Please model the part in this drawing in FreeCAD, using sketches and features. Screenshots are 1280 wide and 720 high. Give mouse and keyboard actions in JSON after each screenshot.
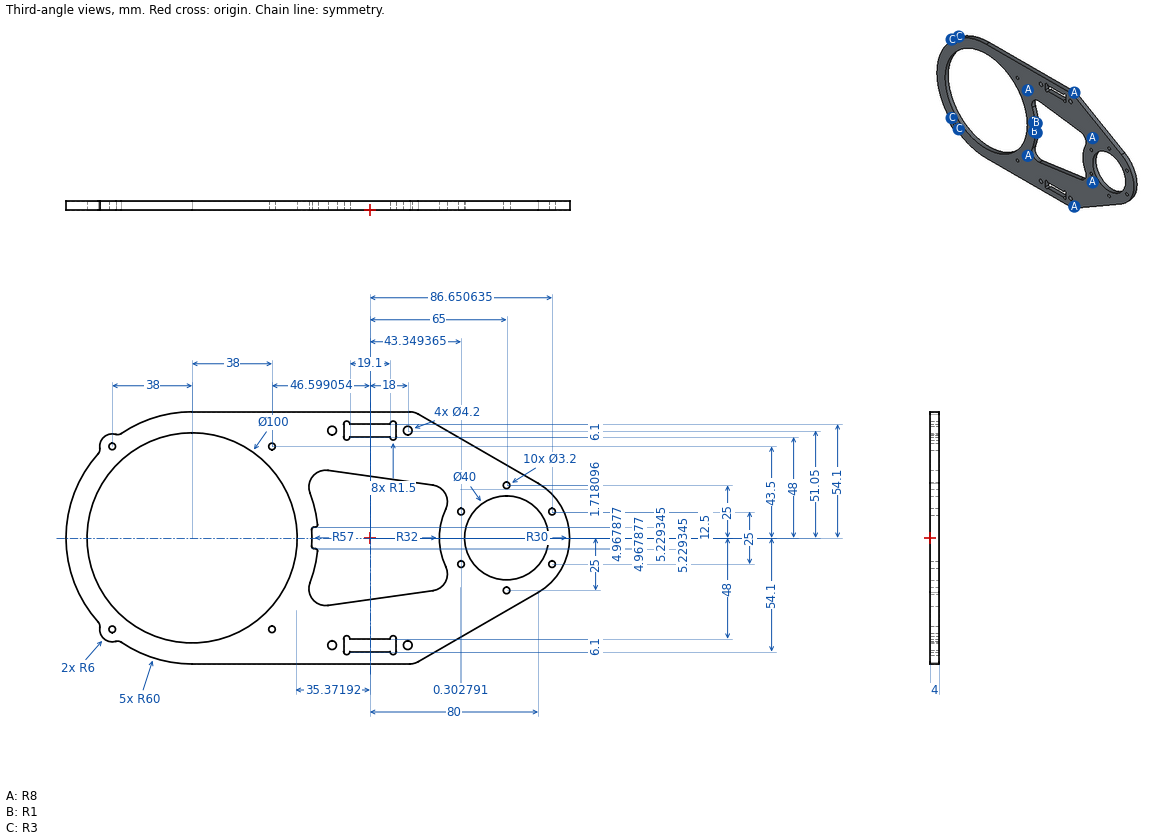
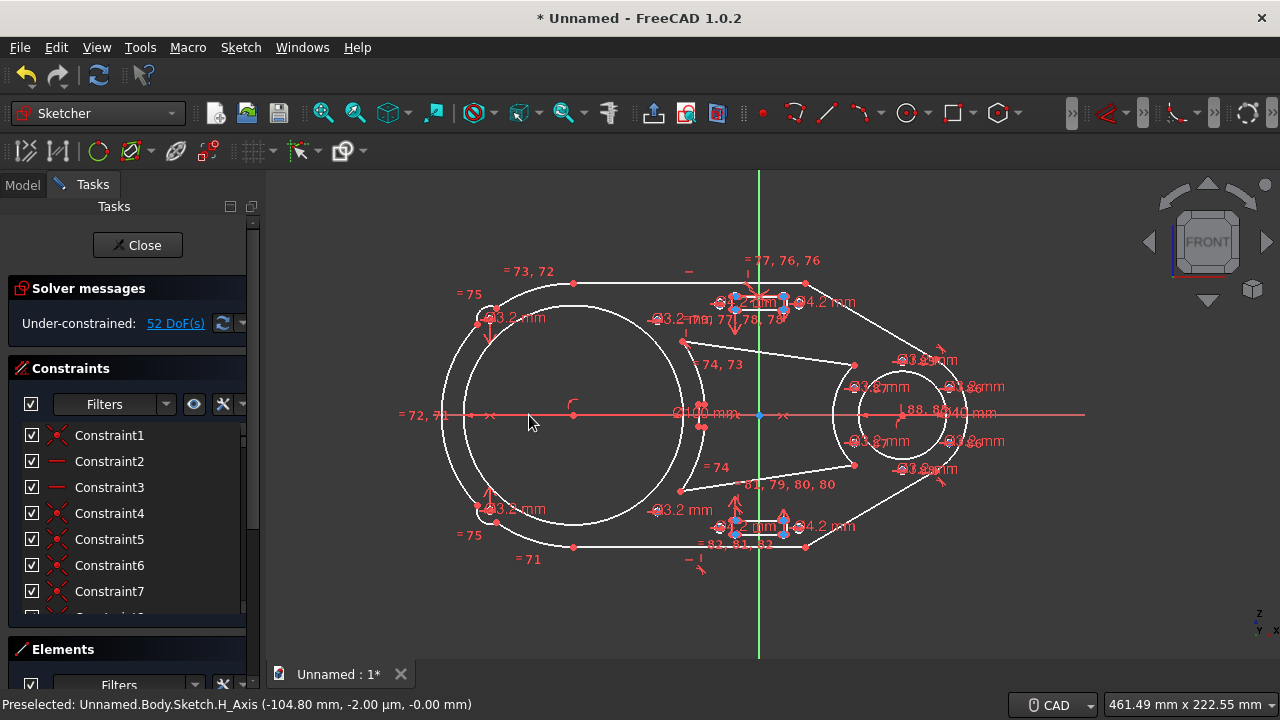
{"action": "left_click", "coordinate": [799, 304]}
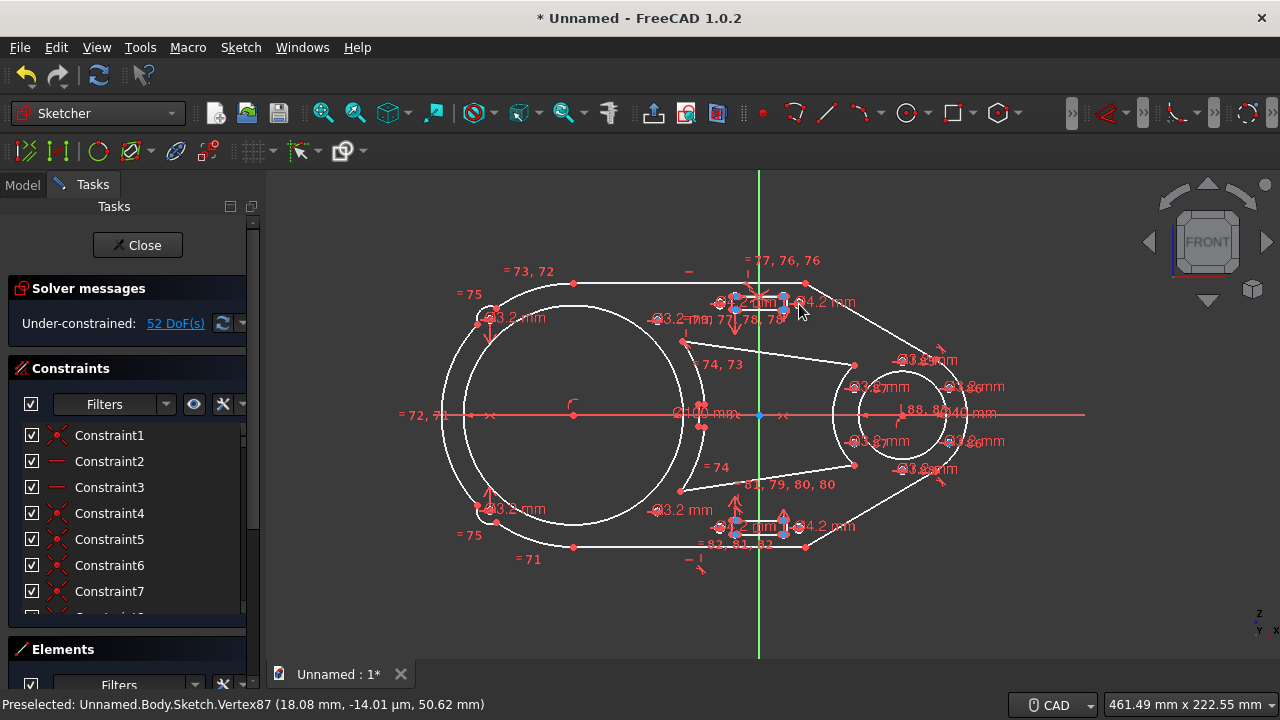
{"action": "left_click", "coordinate": [720, 304]}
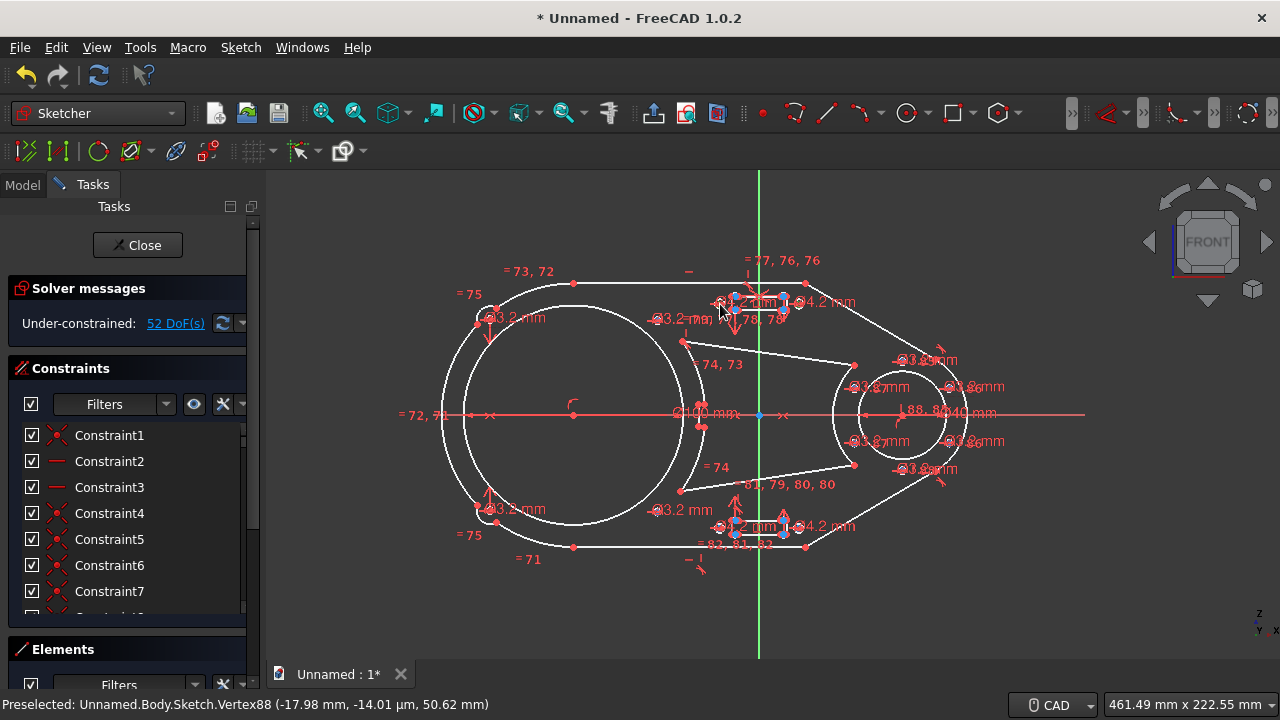
{"action": "left_click", "coordinate": [759, 600]}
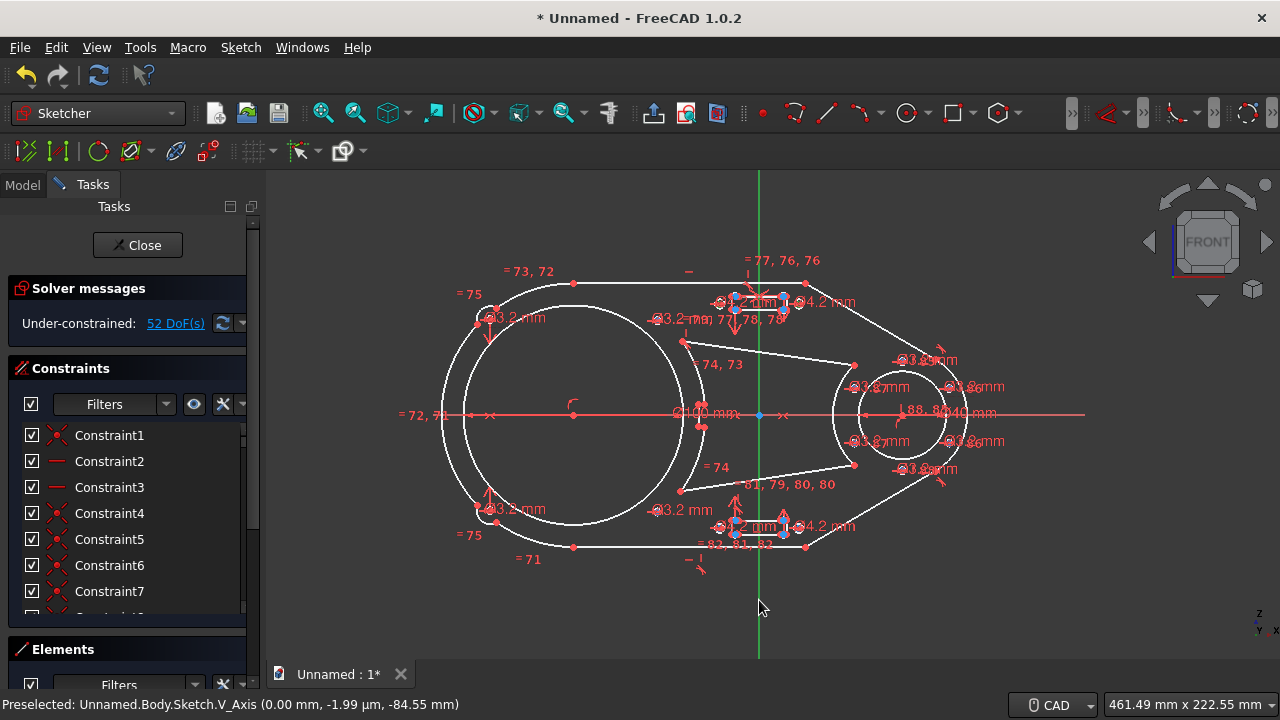
{"action": "key", "text": "s"}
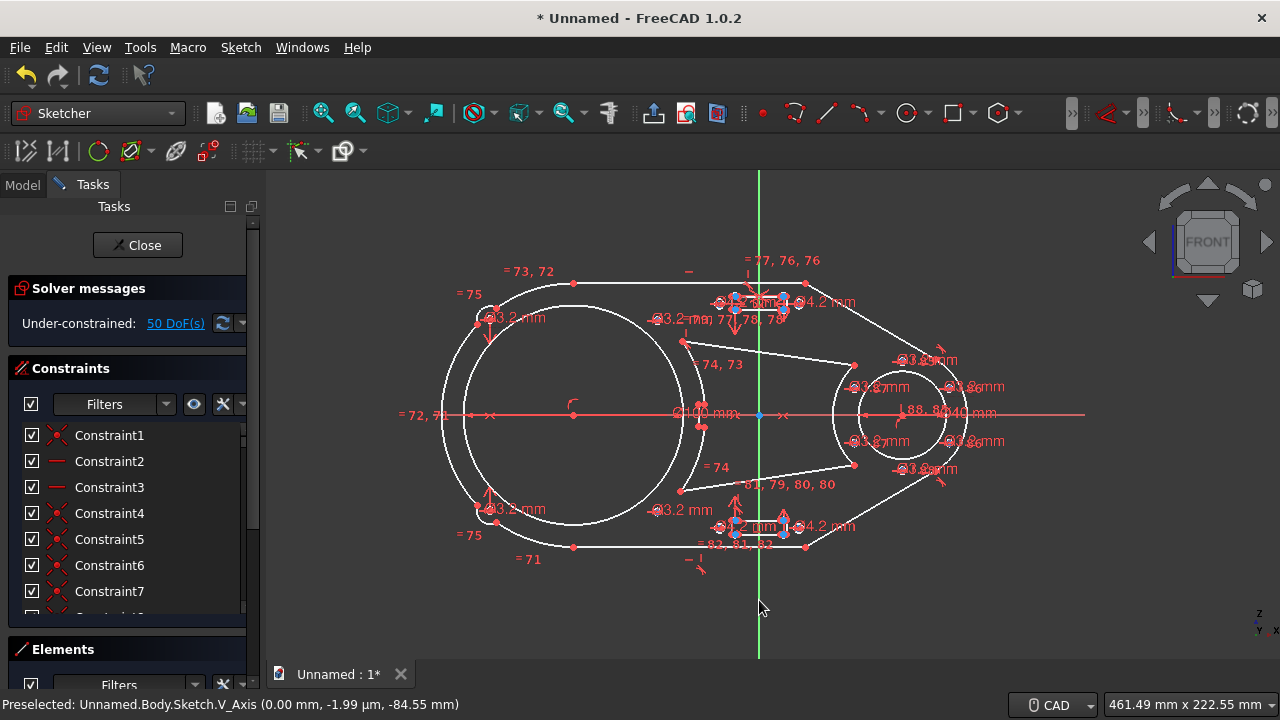
{"action": "left_click", "coordinate": [799, 304]}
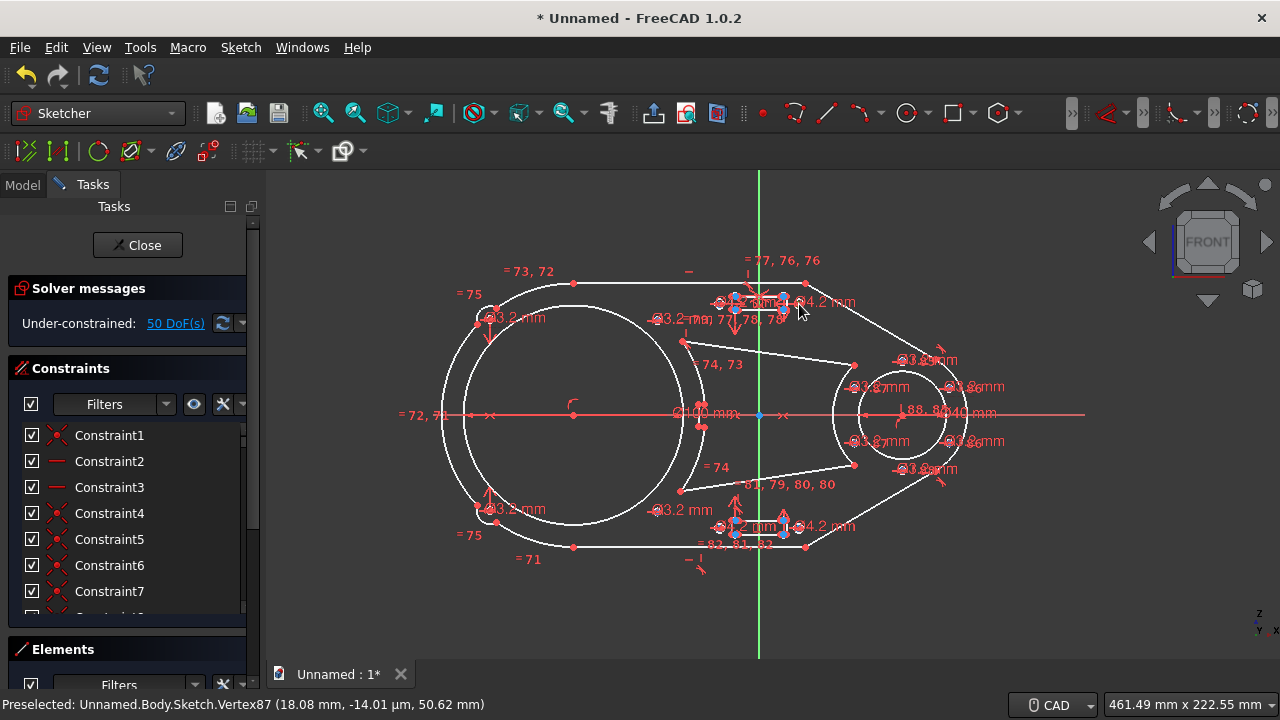
{"action": "left_click", "coordinate": [799, 528]}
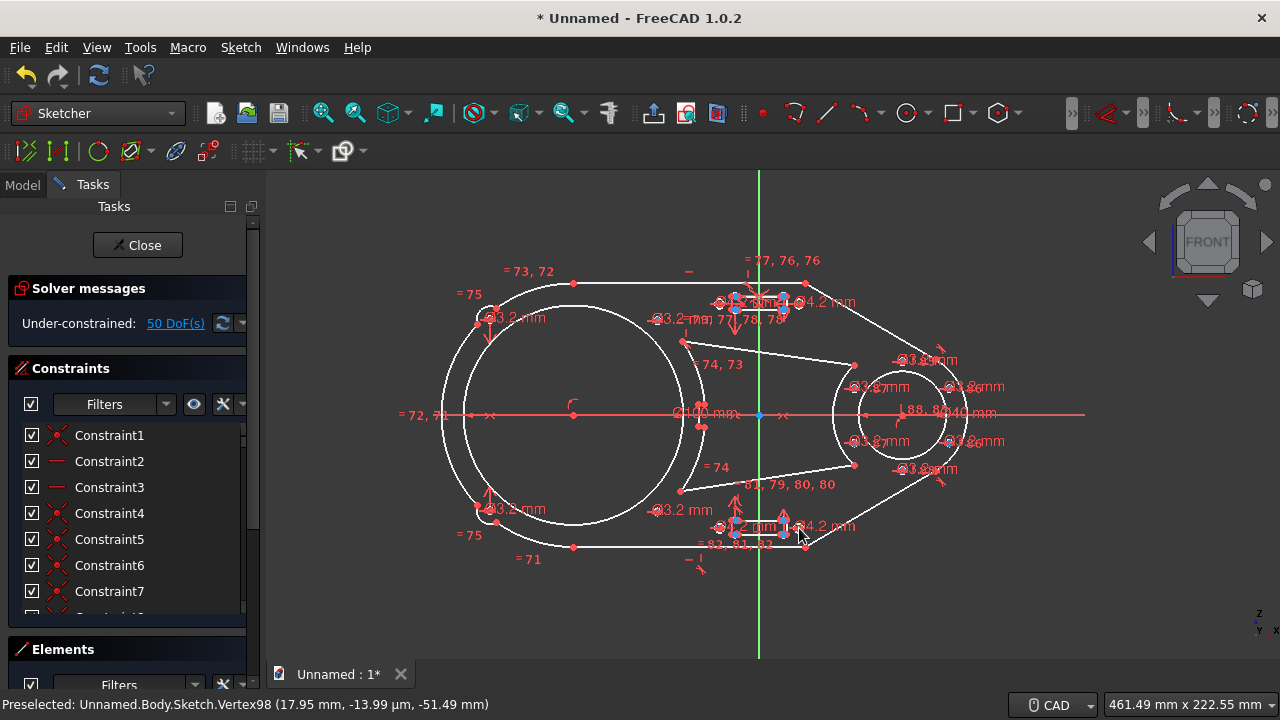
{"action": "left_click", "coordinate": [529, 415]}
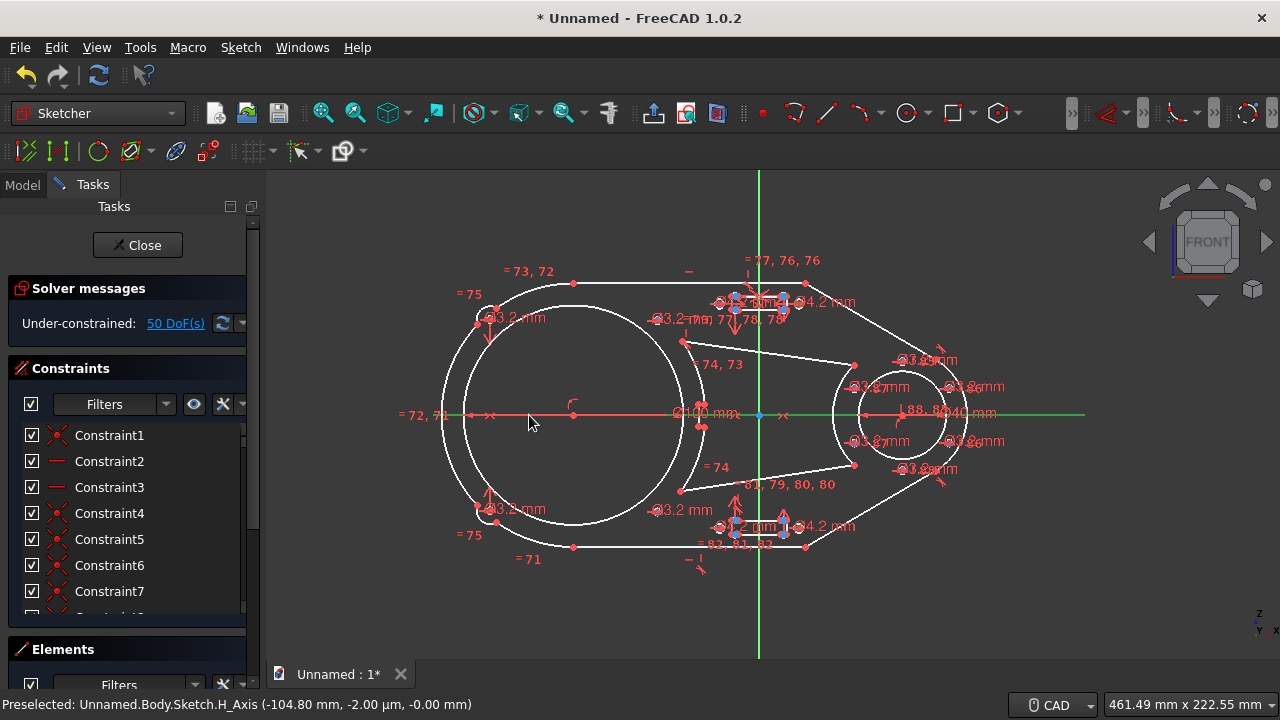
{"action": "key", "text": "s"}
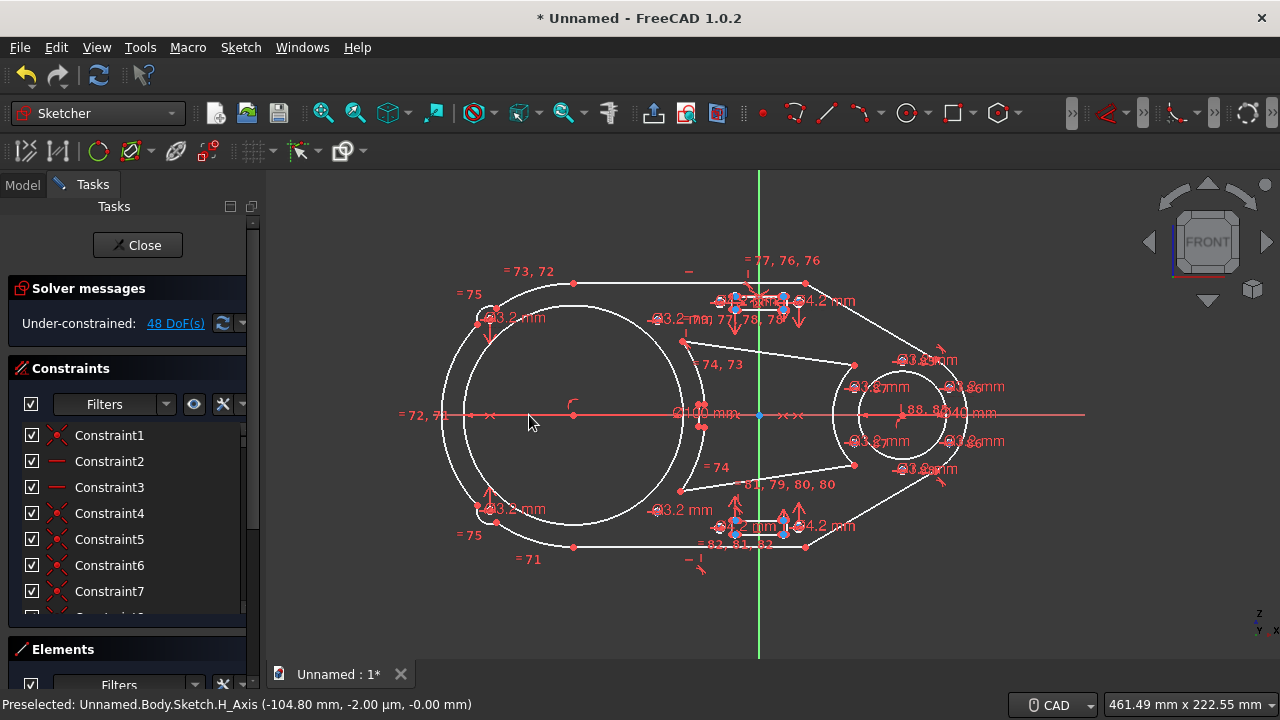
{"action": "left_click", "coordinate": [720, 303]}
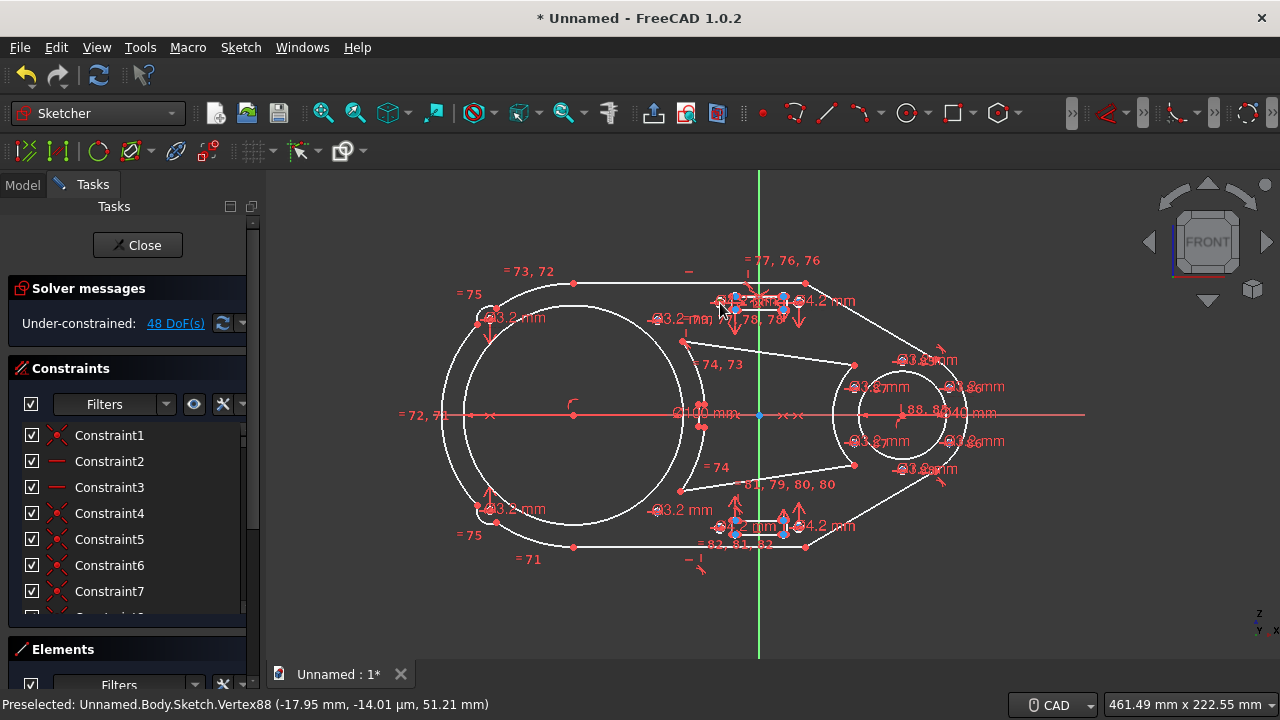
{"action": "left_click", "coordinate": [720, 528]}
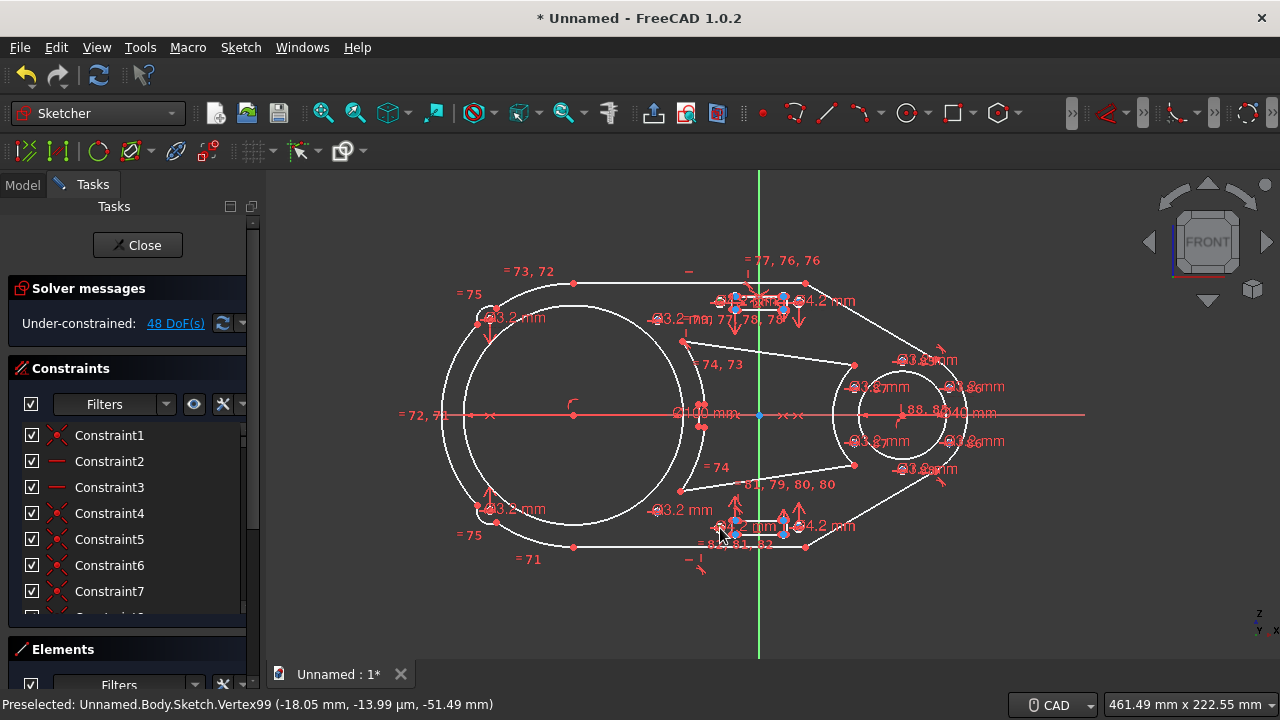
{"action": "left_click", "coordinate": [529, 415]}